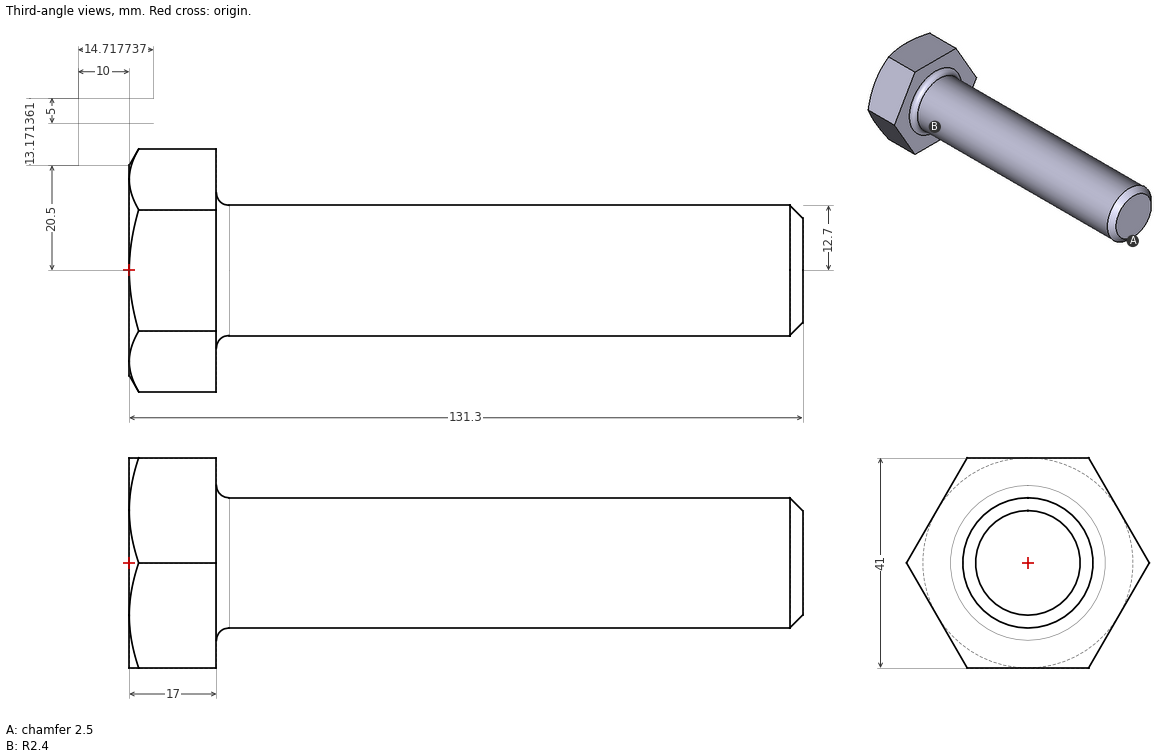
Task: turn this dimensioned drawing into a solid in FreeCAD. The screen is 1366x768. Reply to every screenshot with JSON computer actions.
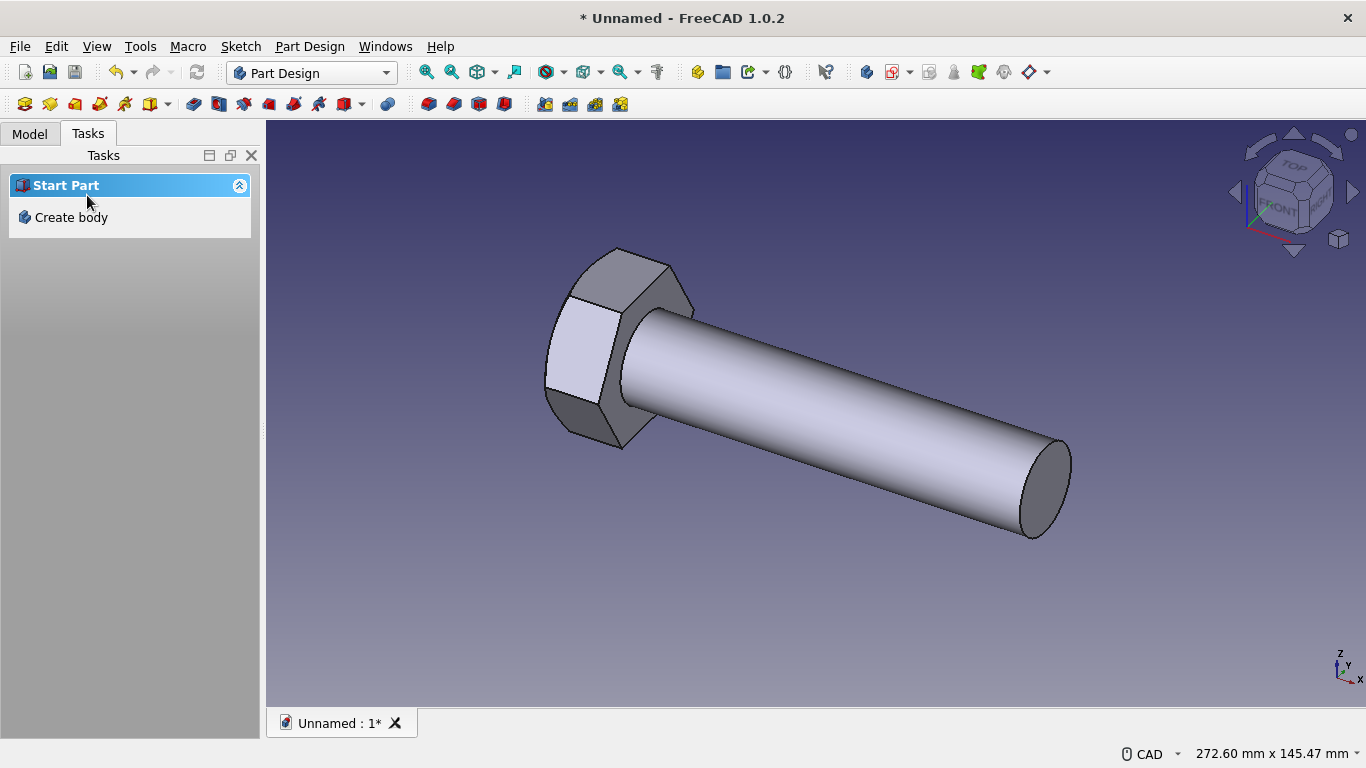
{"action": "left_click", "coordinate": [1020, 514]}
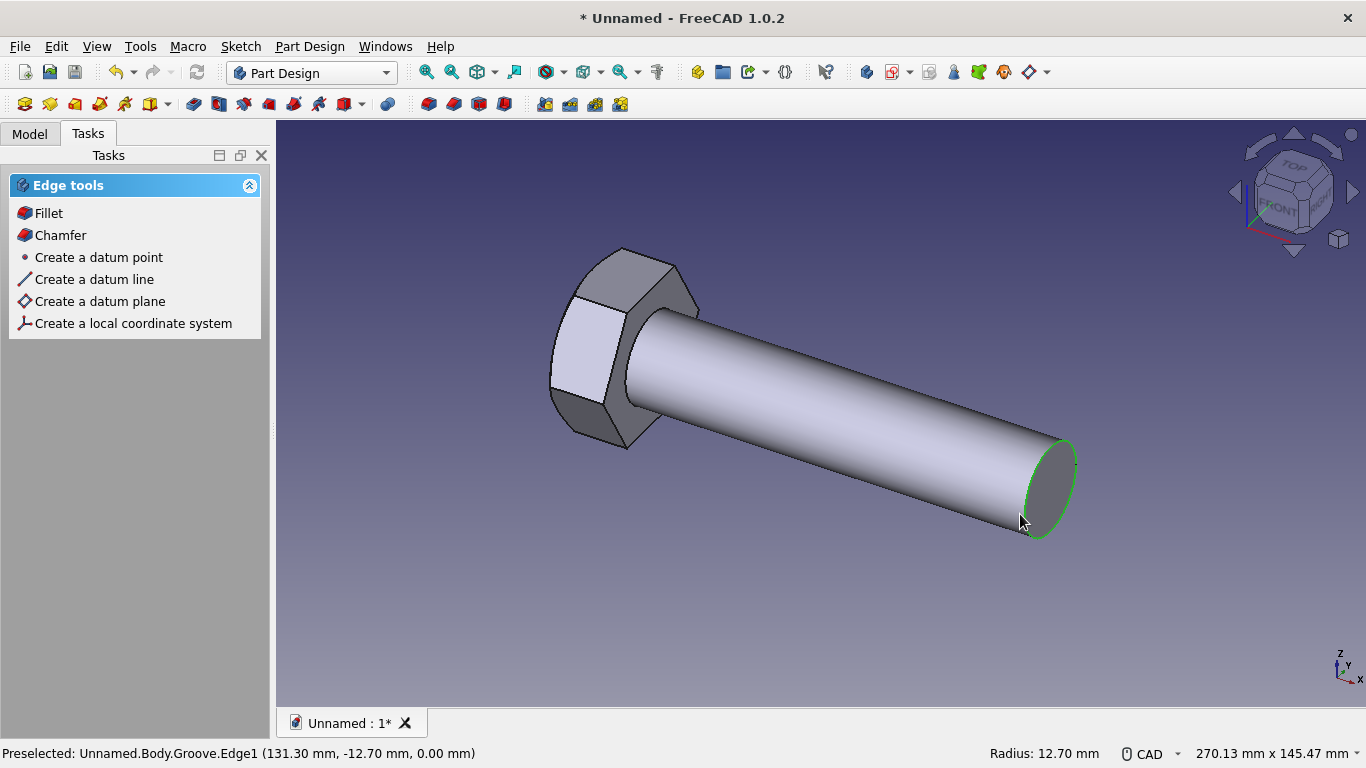
{"action": "left_click", "coordinate": [454, 104]}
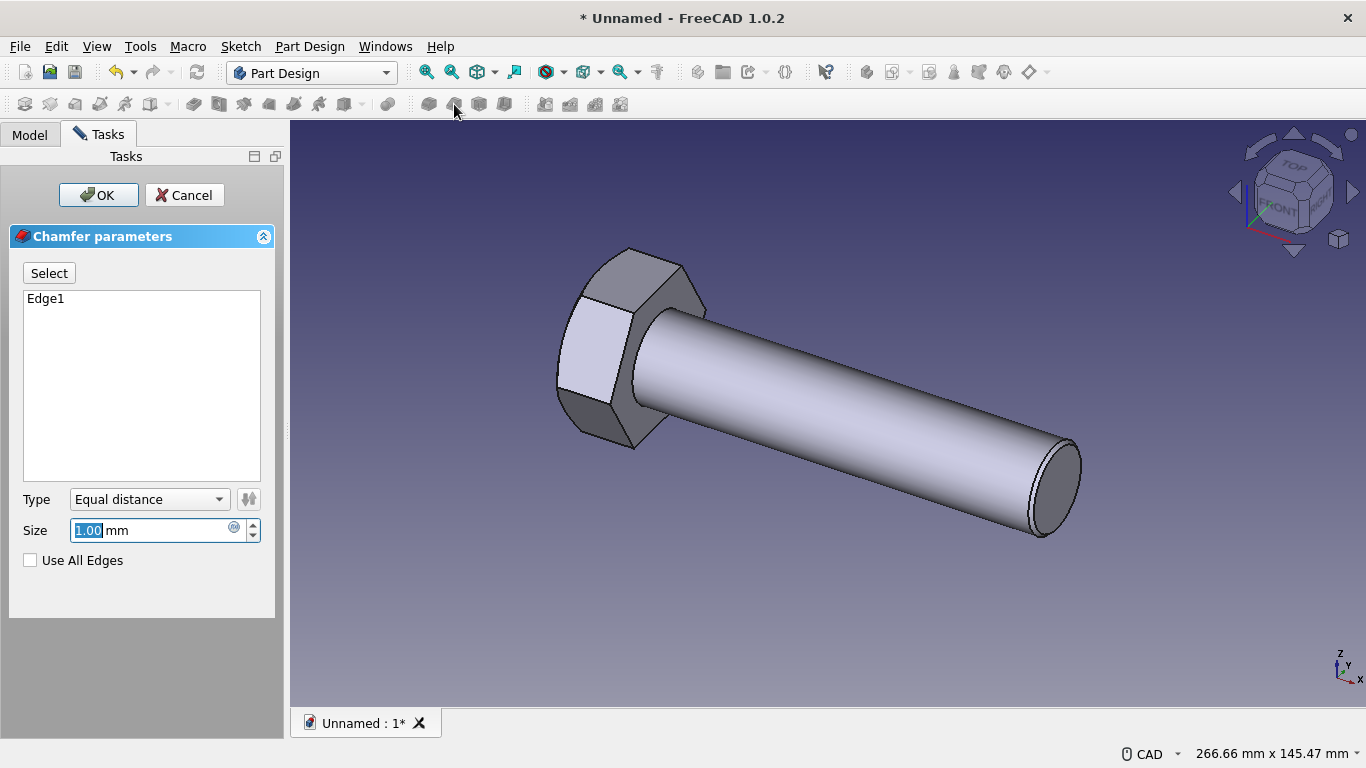
{"action": "type", "text": "2.5"}
{"action": "key", "text": "Tab"}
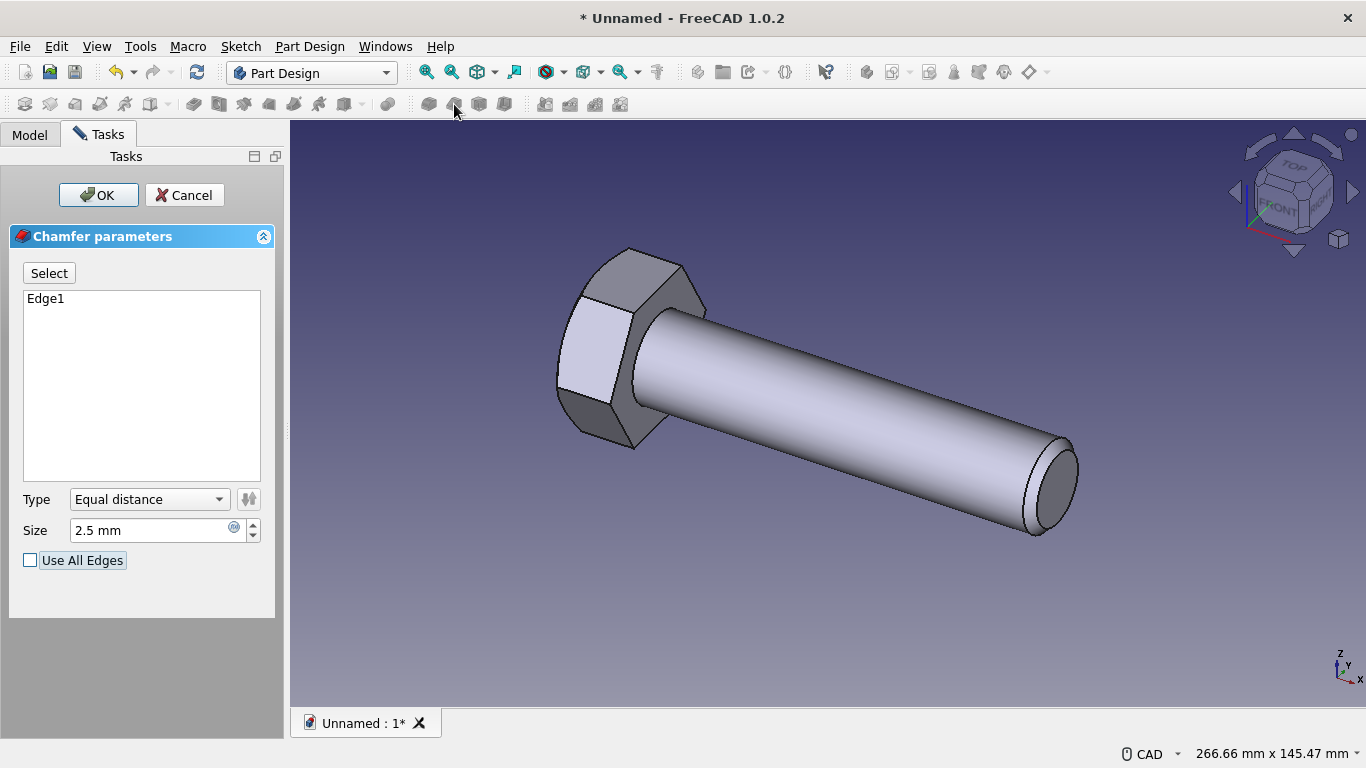
{"action": "left_click", "coordinate": [99, 195]}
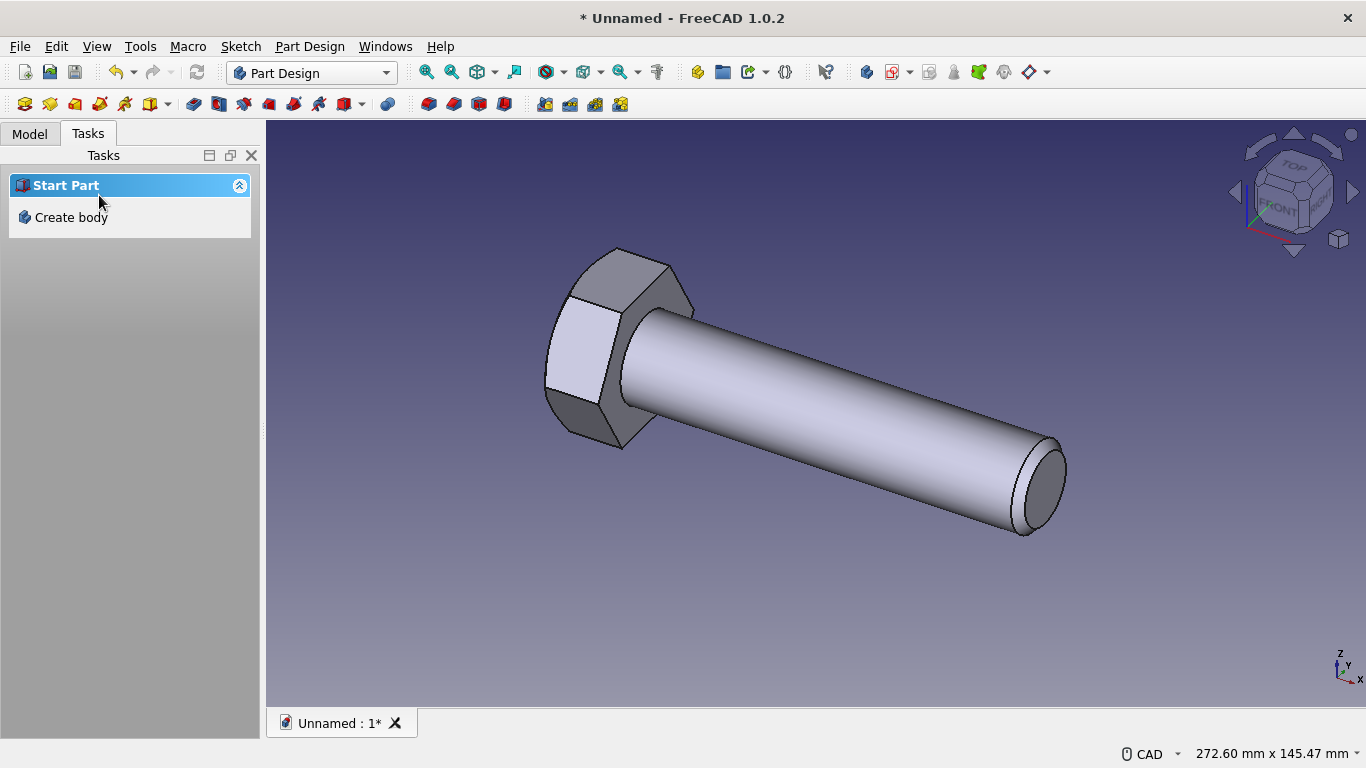
{"action": "key", "text": "0"}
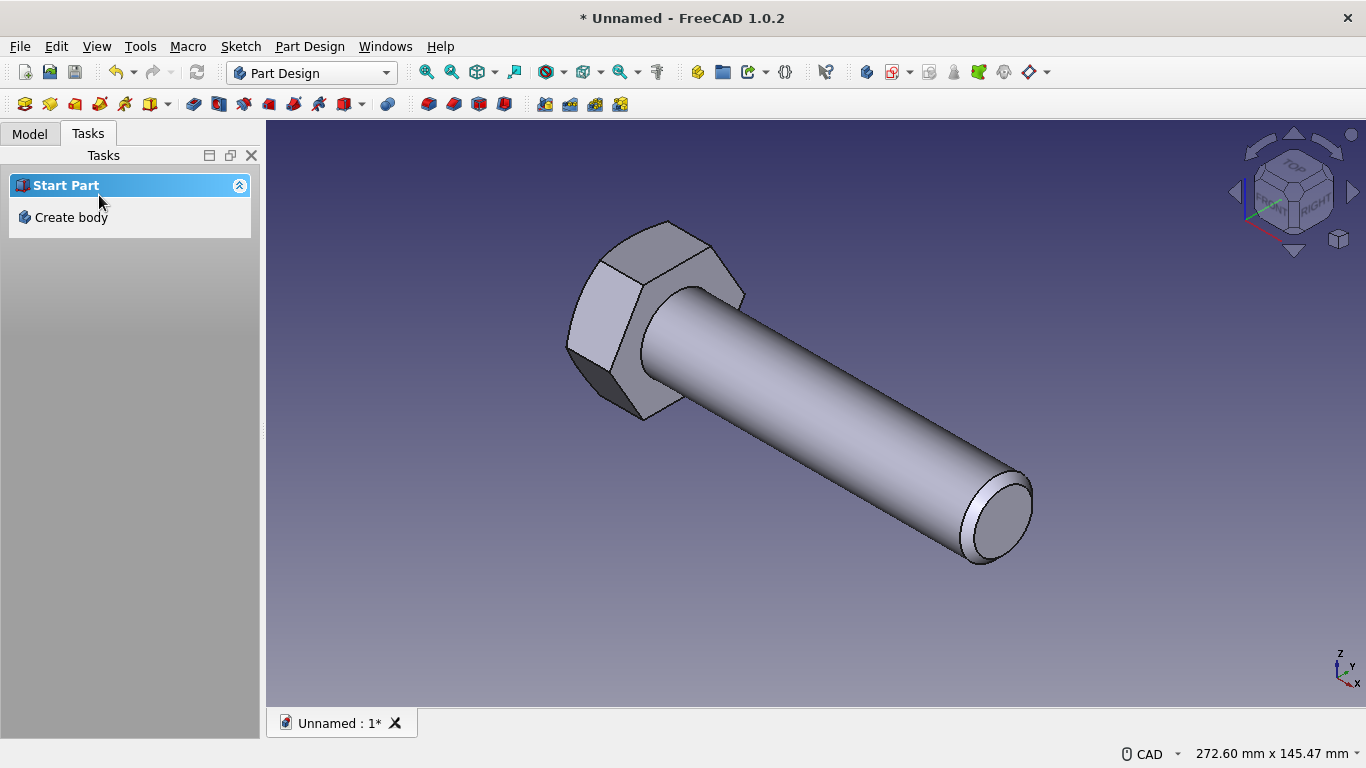
{"action": "key", "text": "2"}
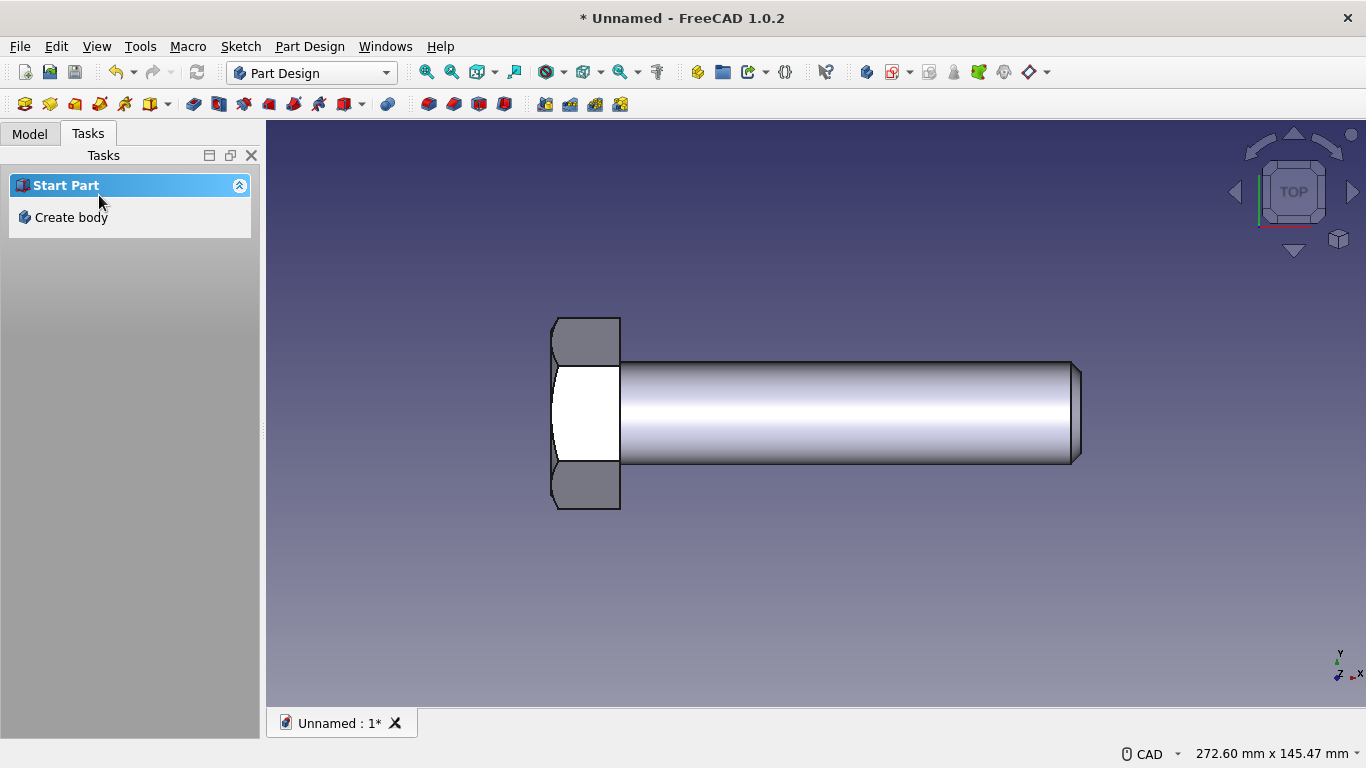
{"action": "key", "text": "1"}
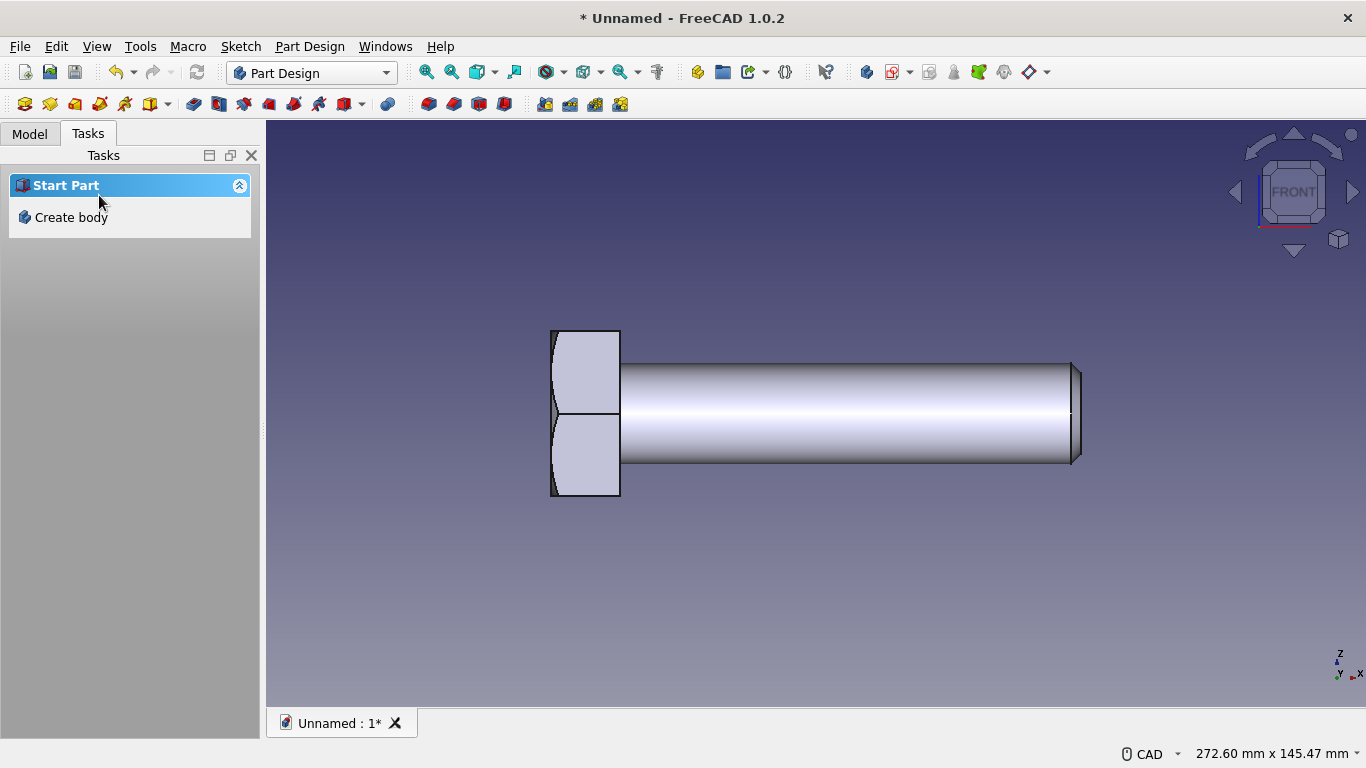
{"action": "key", "text": "3"}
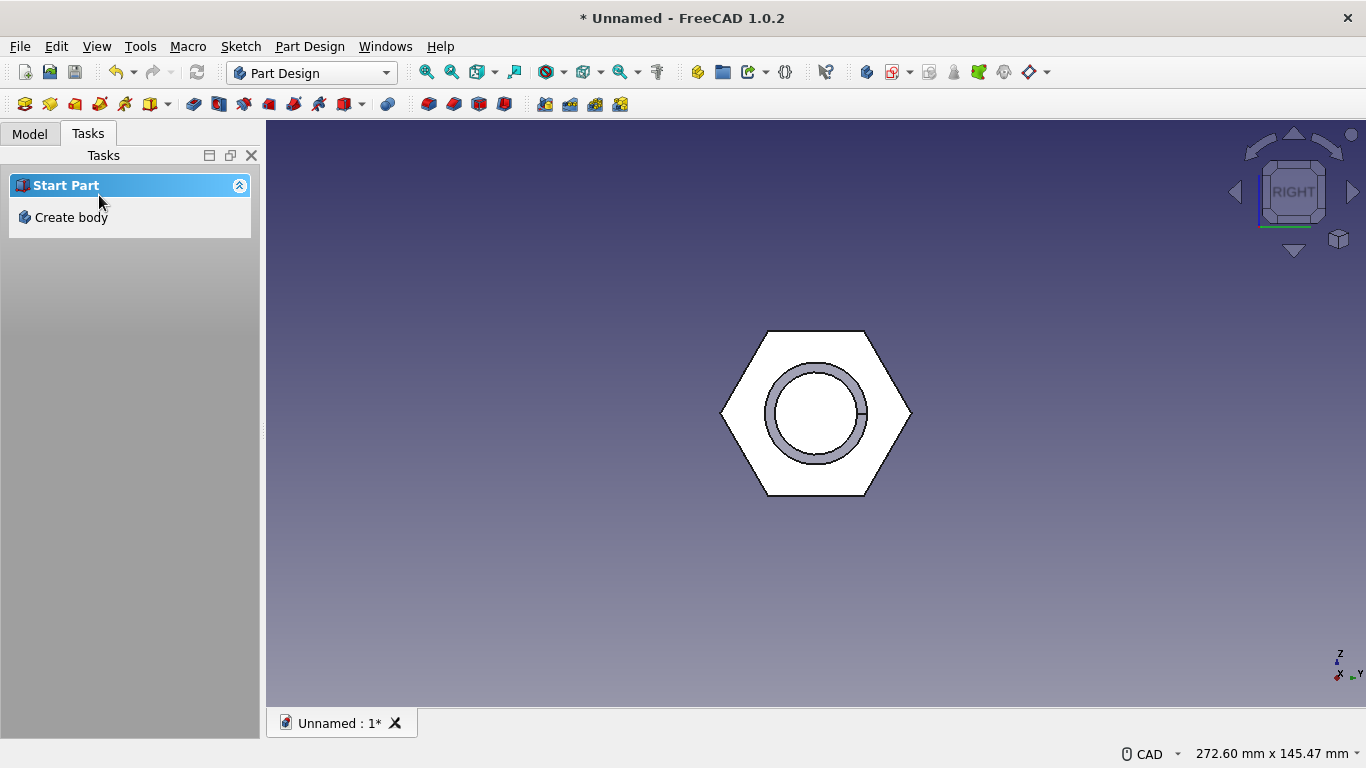
{"action": "key", "text": "v f"}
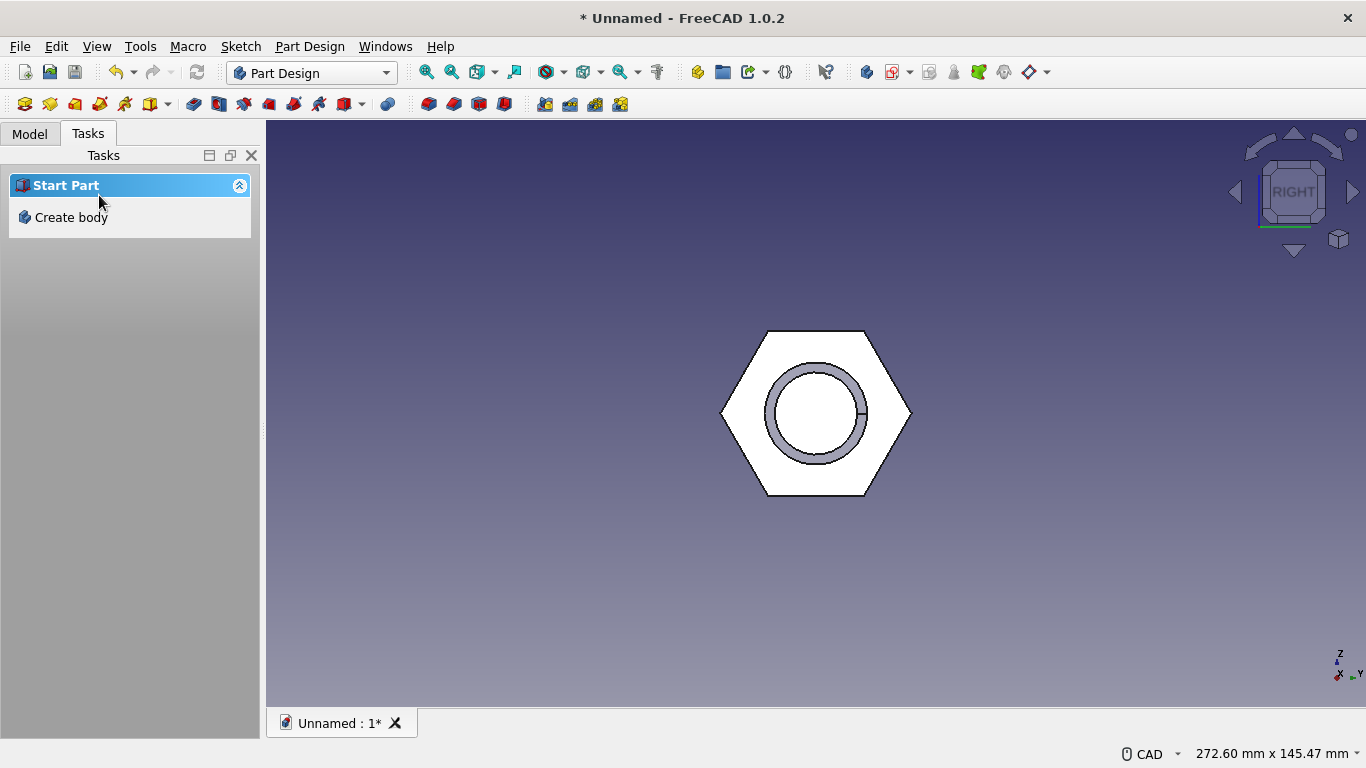
{"action": "key", "text": "5"}